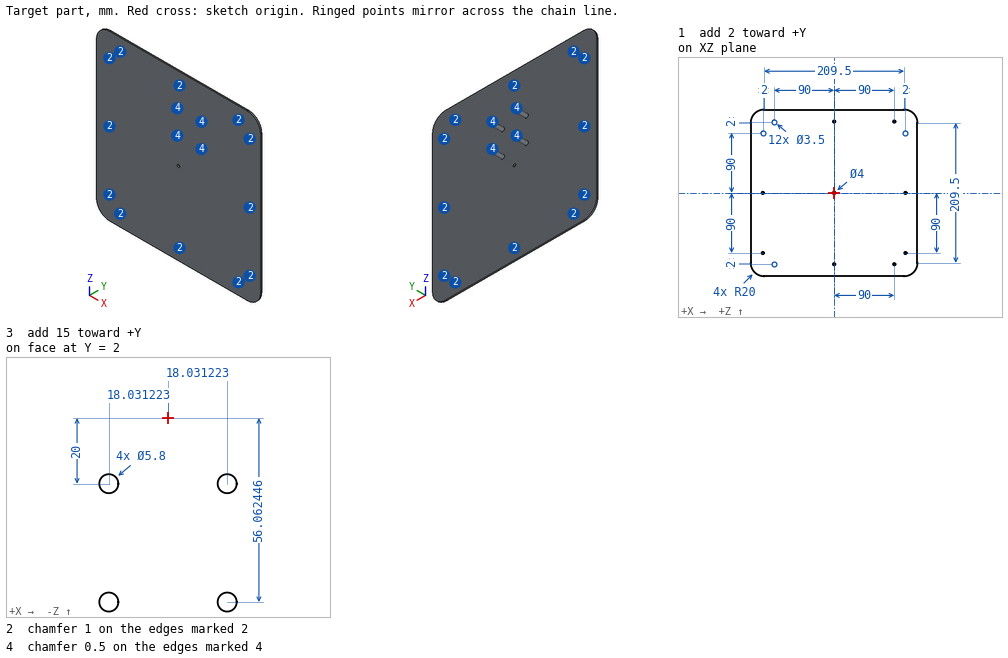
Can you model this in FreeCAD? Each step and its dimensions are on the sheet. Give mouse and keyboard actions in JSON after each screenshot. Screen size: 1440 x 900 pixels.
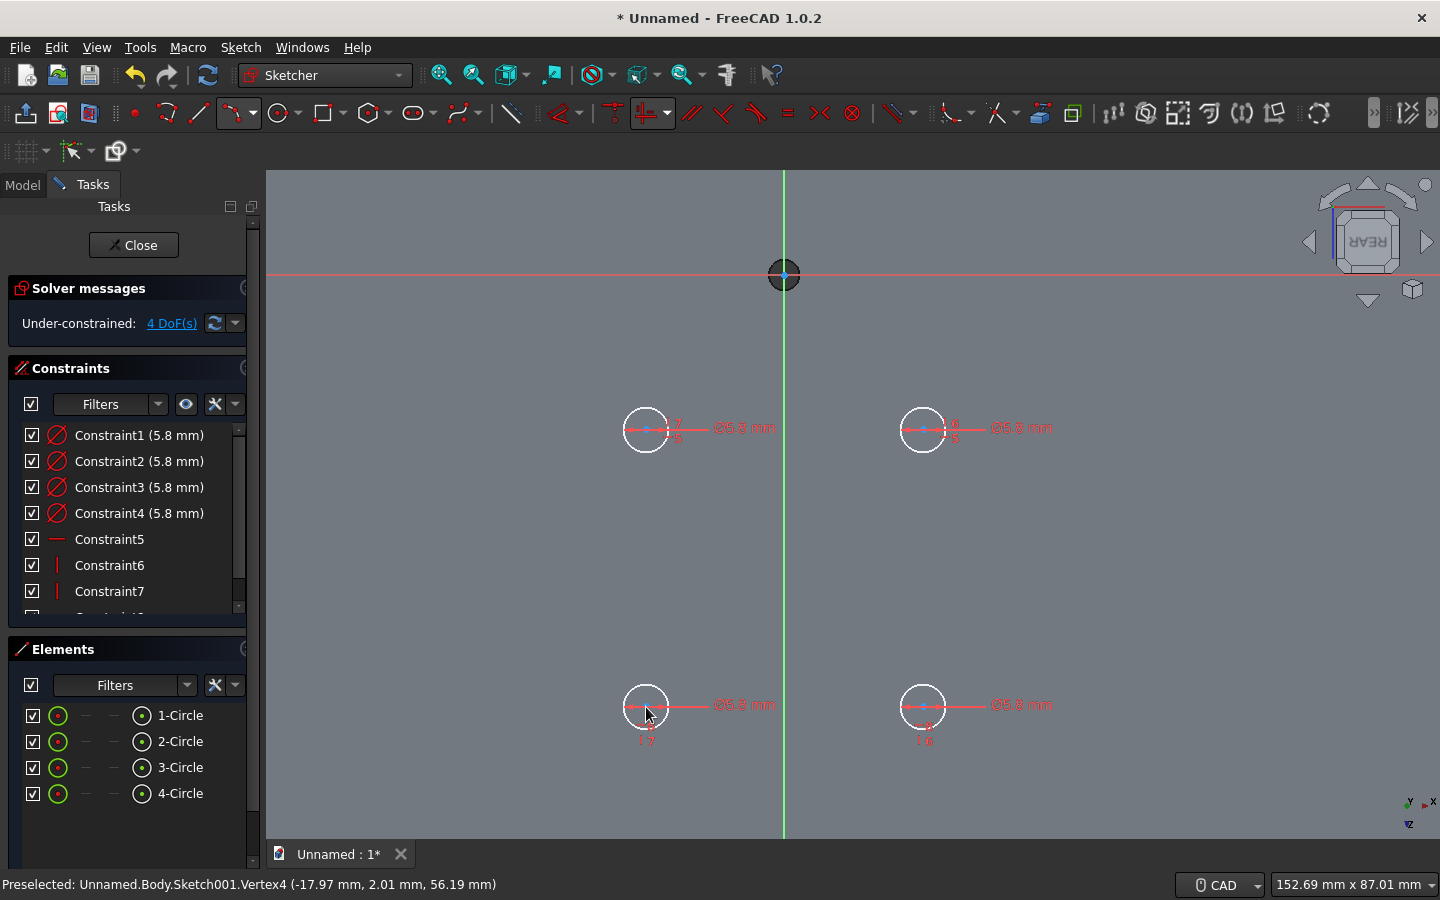
{"action": "left_click", "coordinate": [558, 114]}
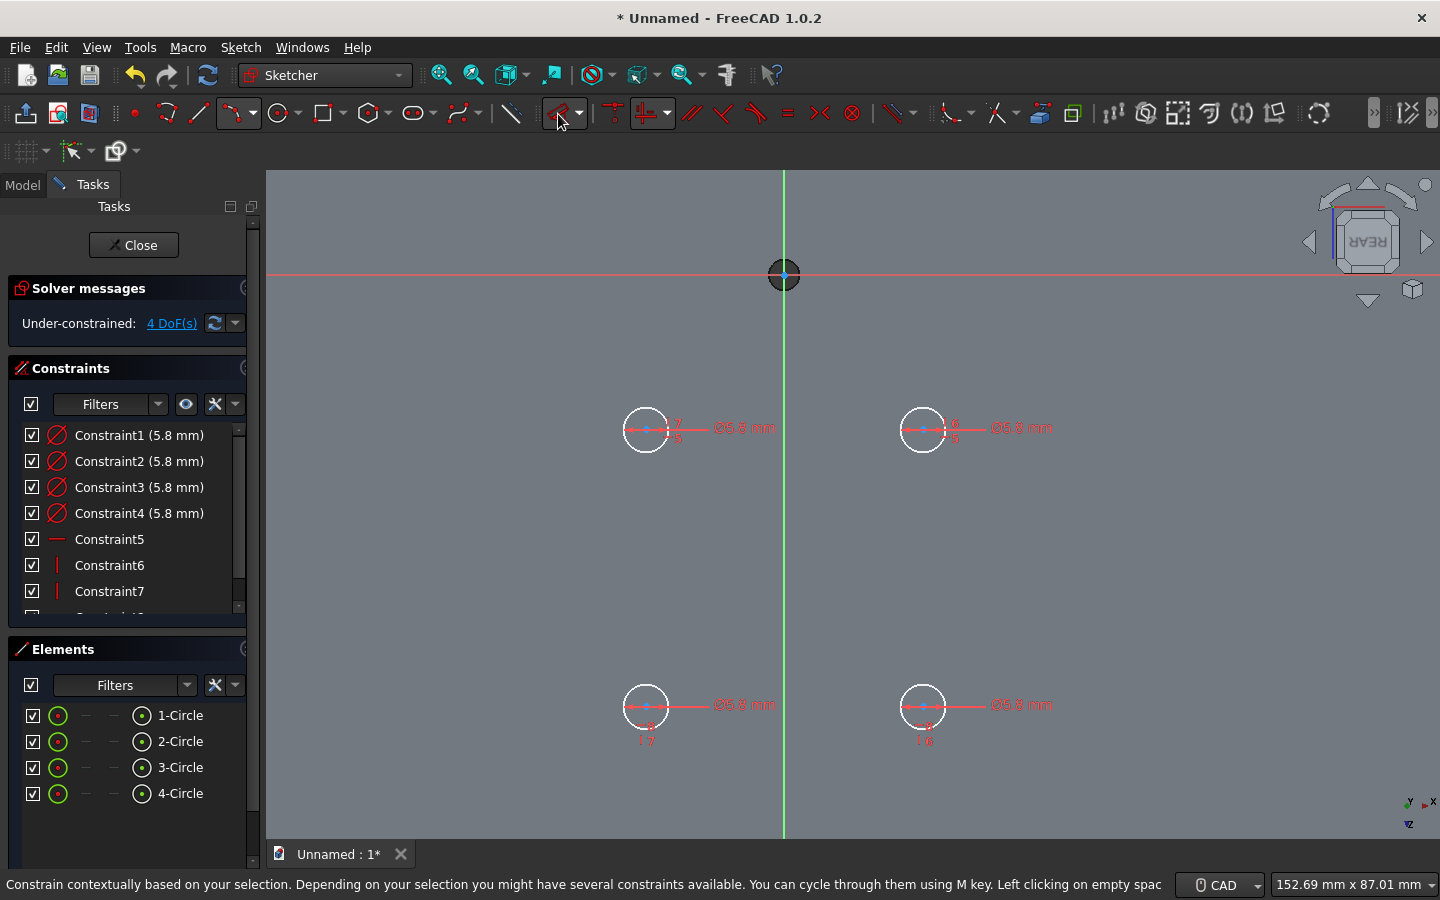
{"action": "left_click", "coordinate": [646, 430]}
{"action": "left_click", "coordinate": [612, 353]}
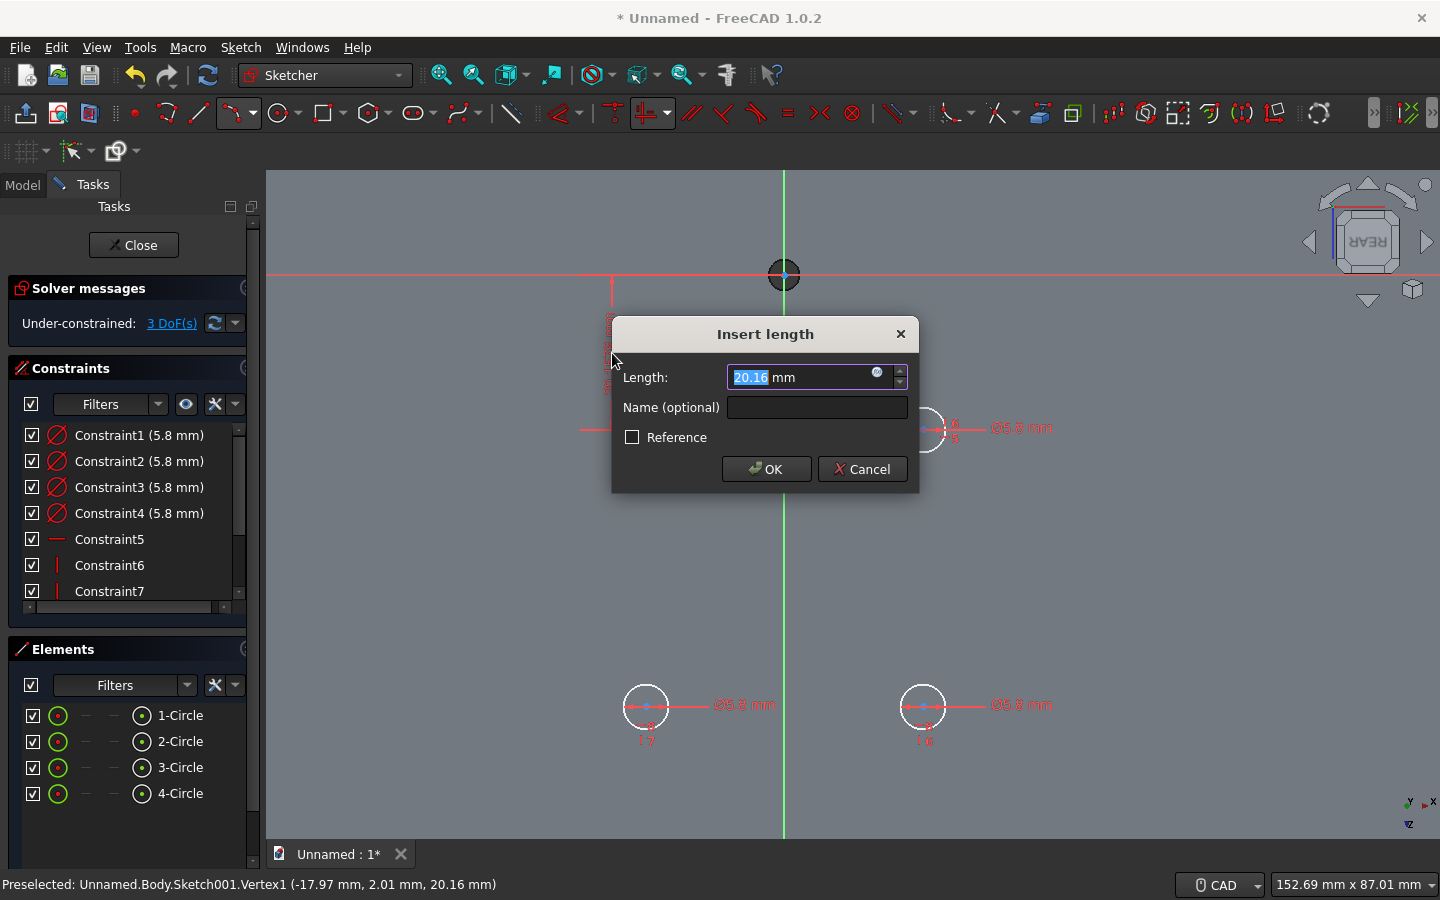
{"action": "type", "text": "20"}
{"action": "key", "text": "Return"}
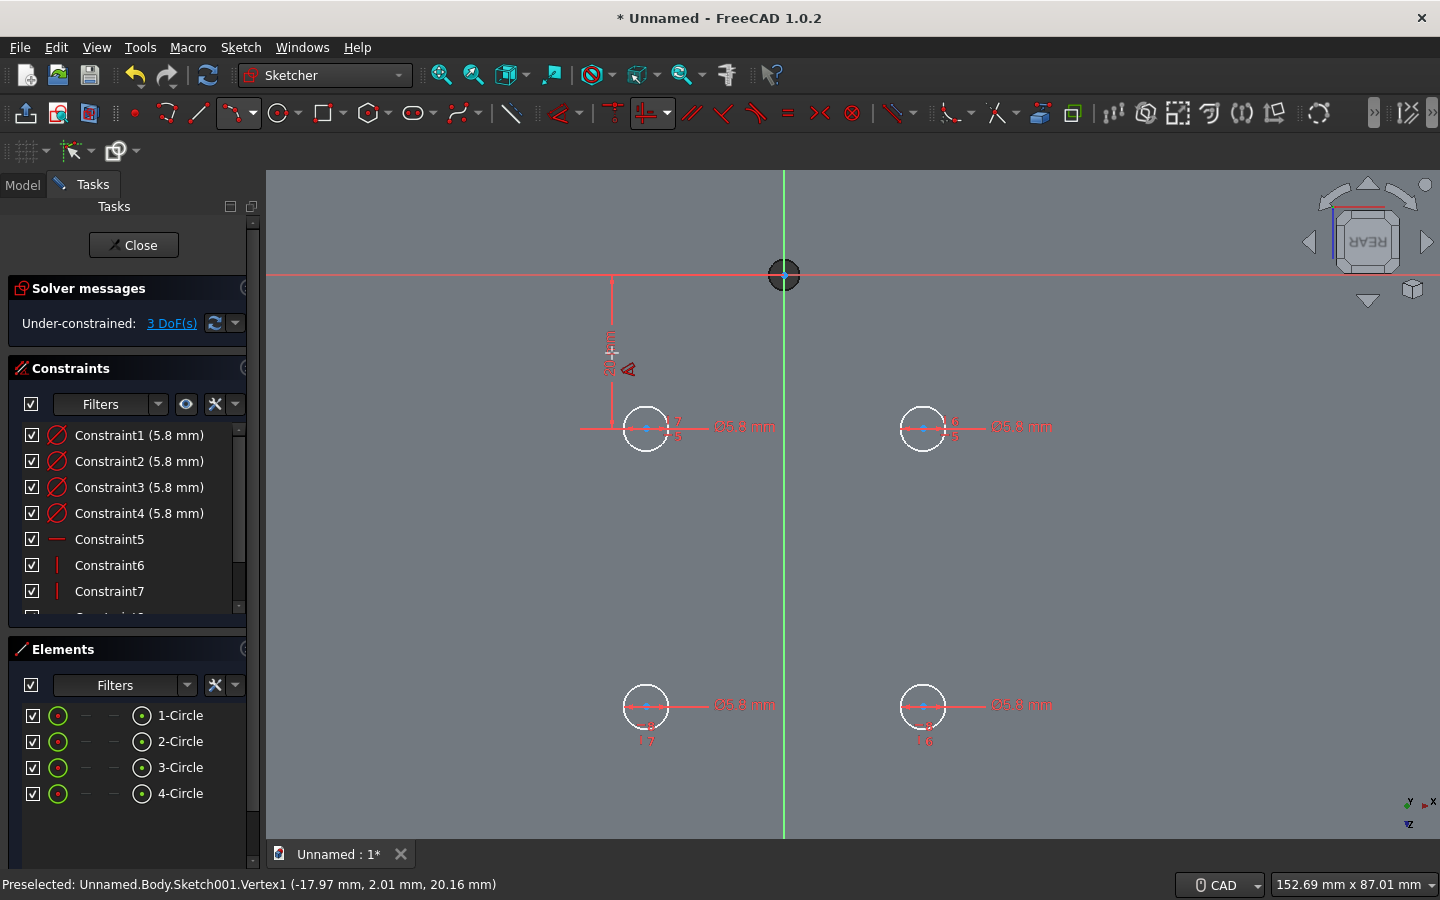
{"action": "left_click", "coordinate": [646, 429]}
{"action": "left_click", "coordinate": [715, 241]}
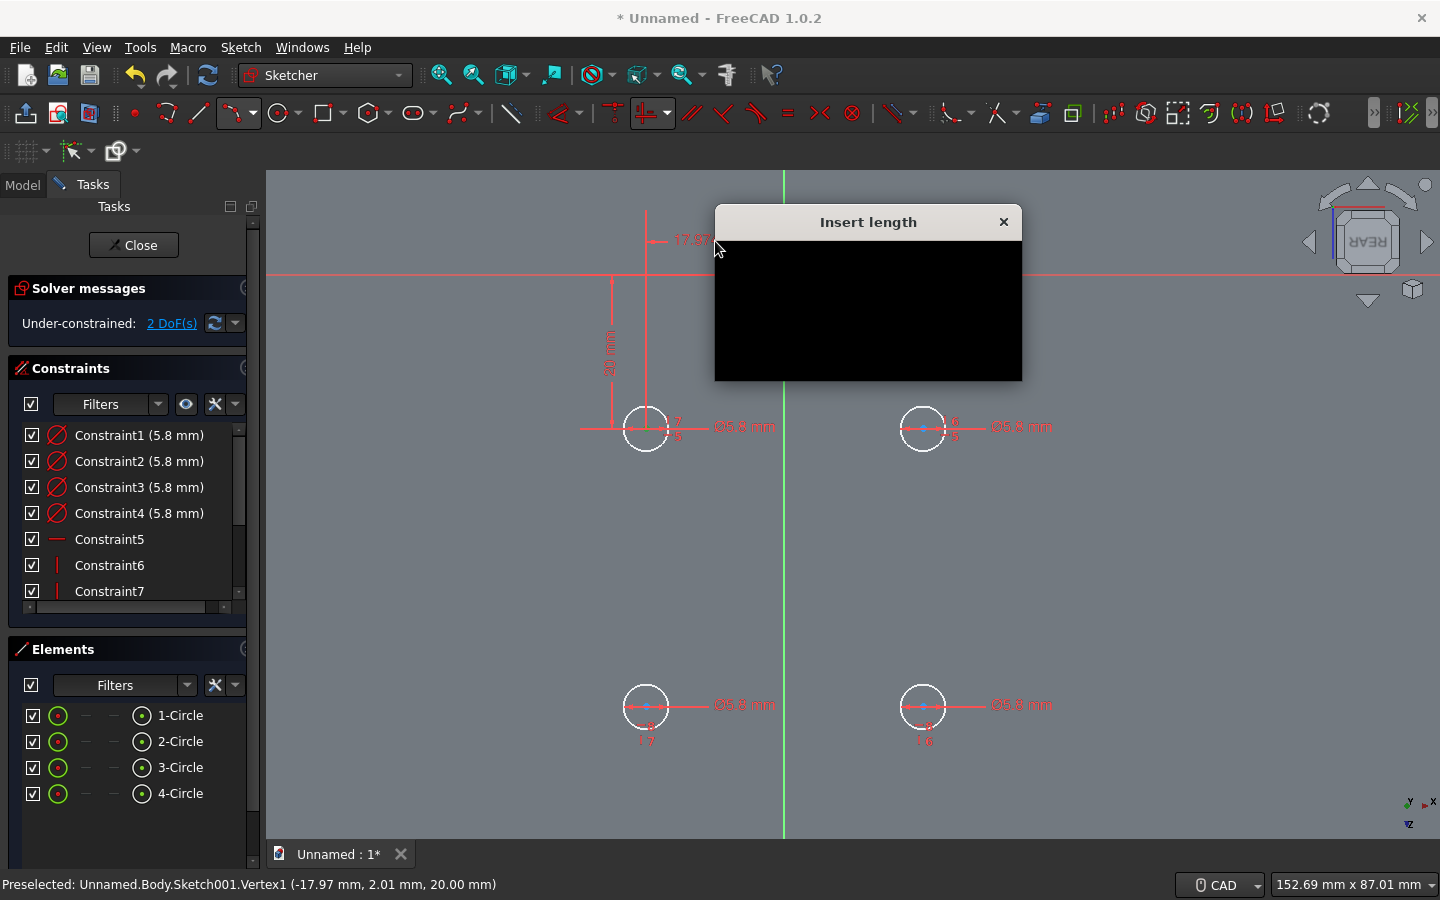
{"action": "type", "text": "18.031223"}
{"action": "key", "text": "Return"}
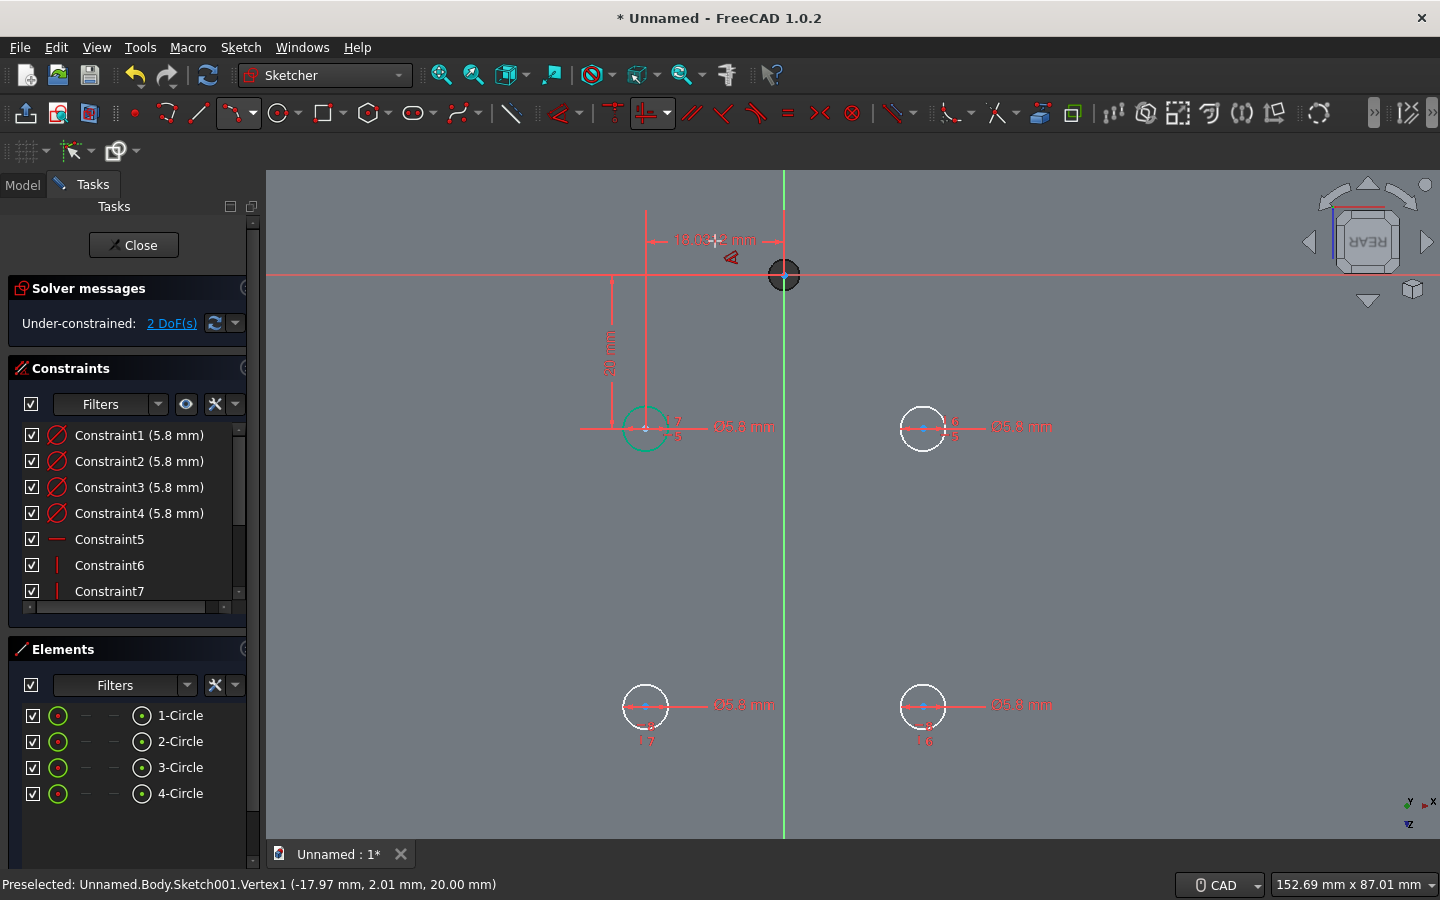
{"action": "left_click", "coordinate": [923, 429]}
{"action": "left_click", "coordinate": [854, 241]}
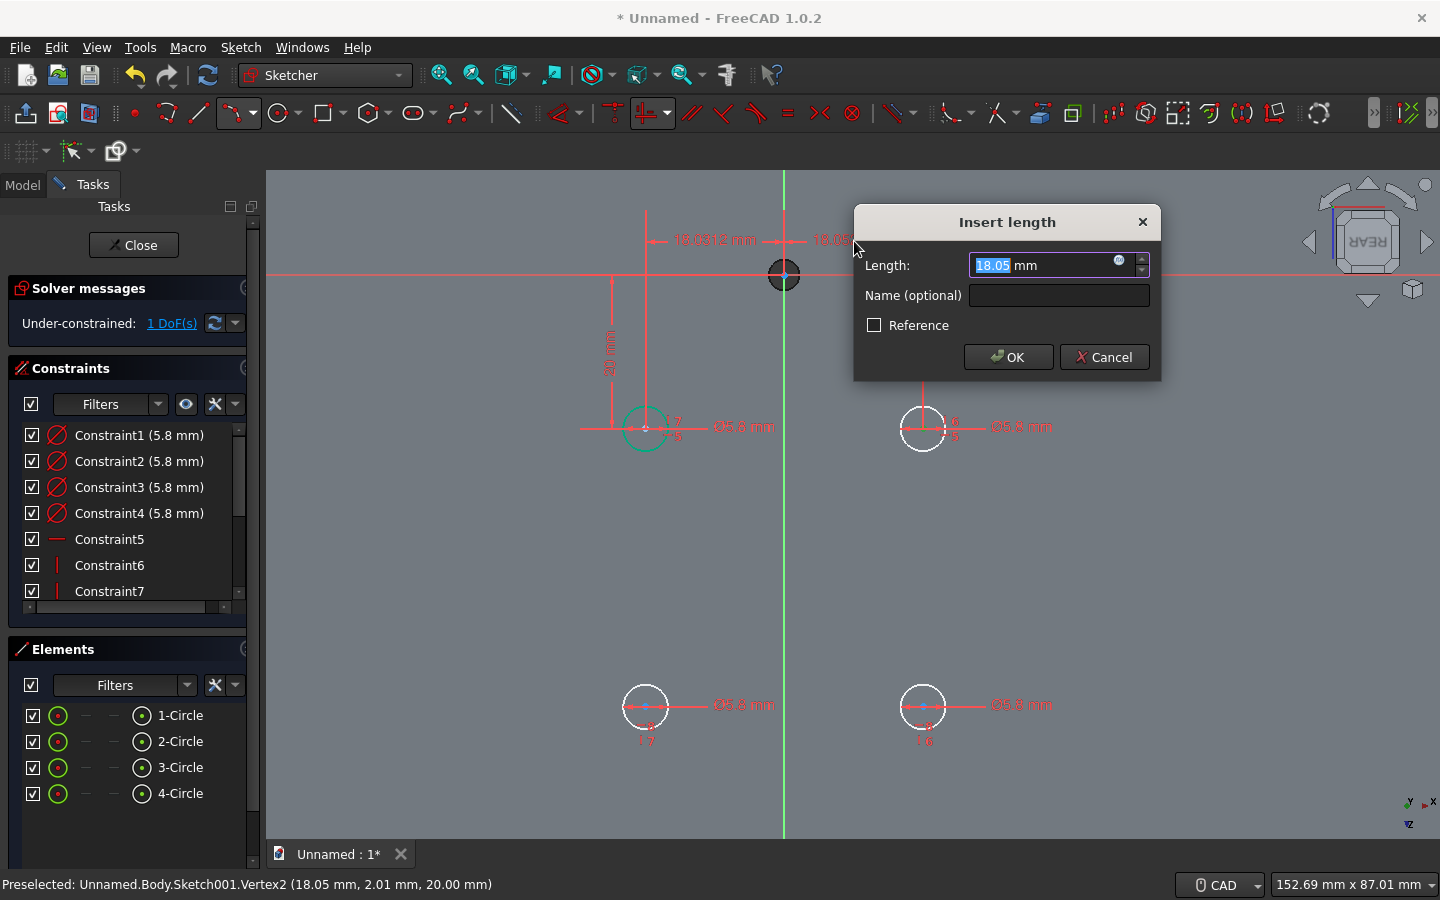
{"action": "type", "text": "18.031223"}
{"action": "key", "text": "Return"}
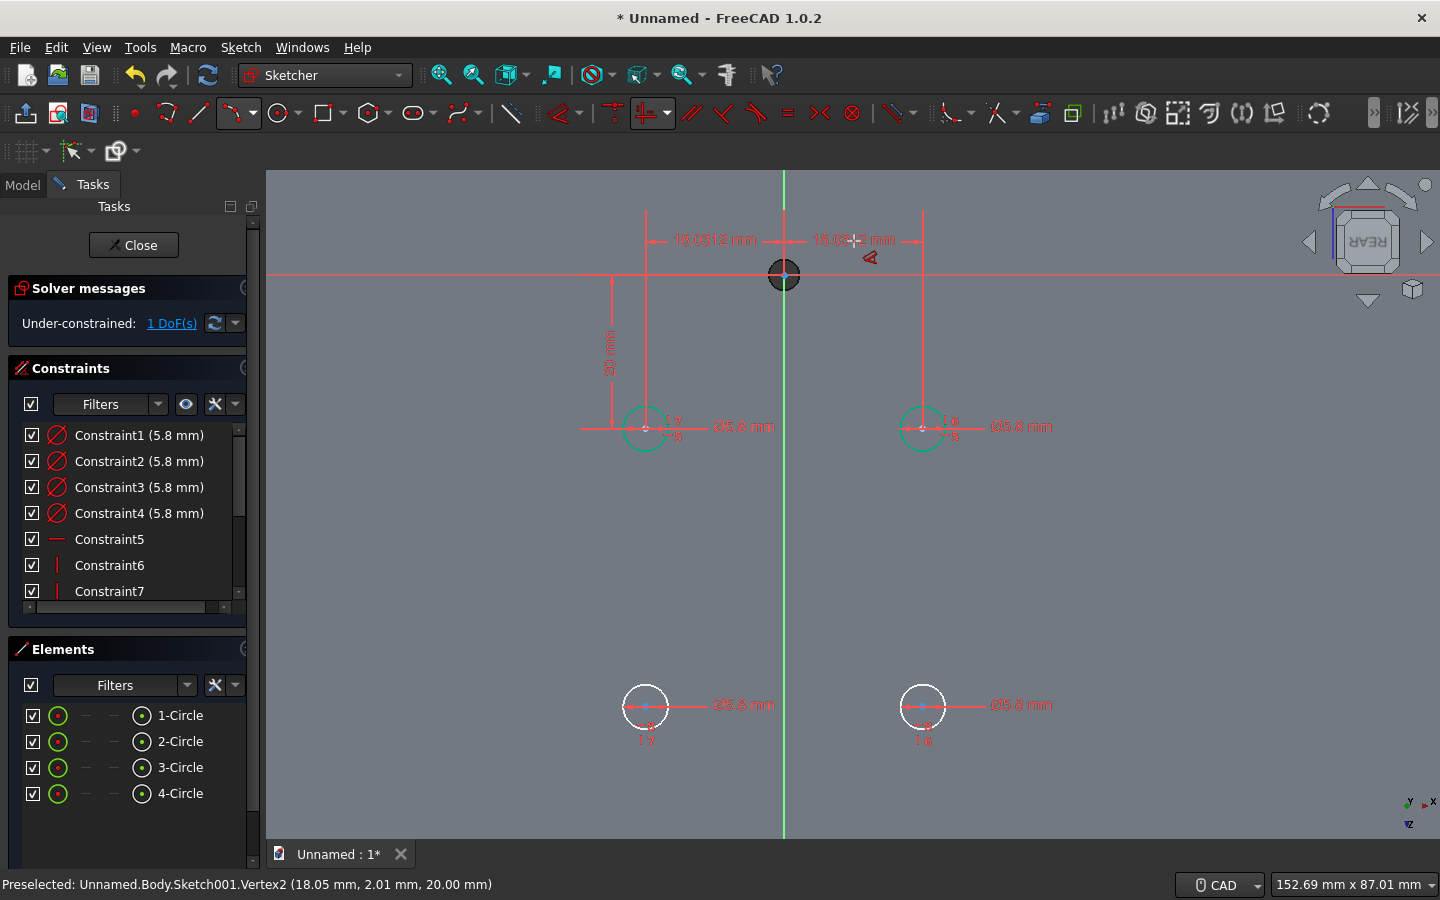
{"action": "left_click", "coordinate": [923, 707]}
{"action": "left_click", "coordinate": [957, 491]}